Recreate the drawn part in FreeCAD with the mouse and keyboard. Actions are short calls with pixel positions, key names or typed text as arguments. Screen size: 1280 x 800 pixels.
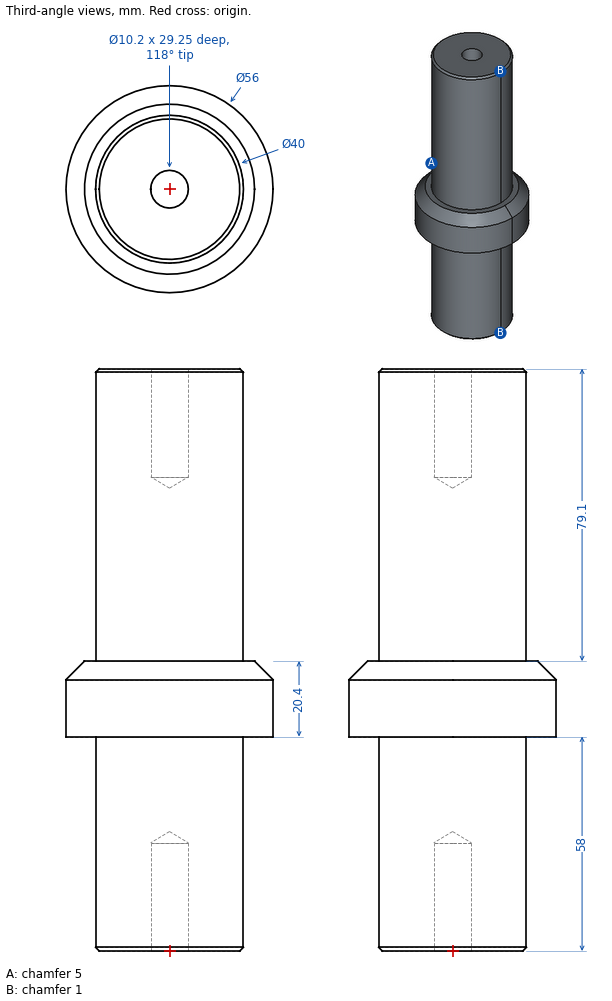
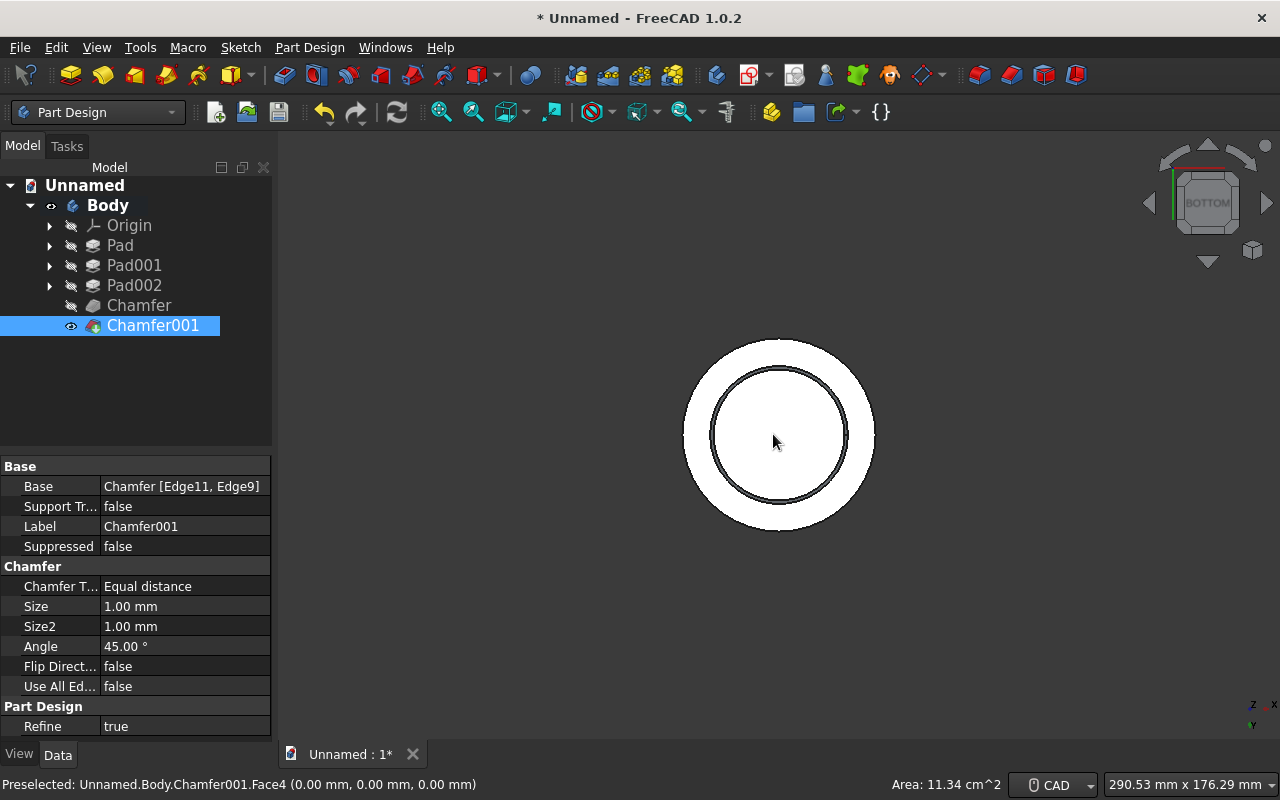
click(750, 76)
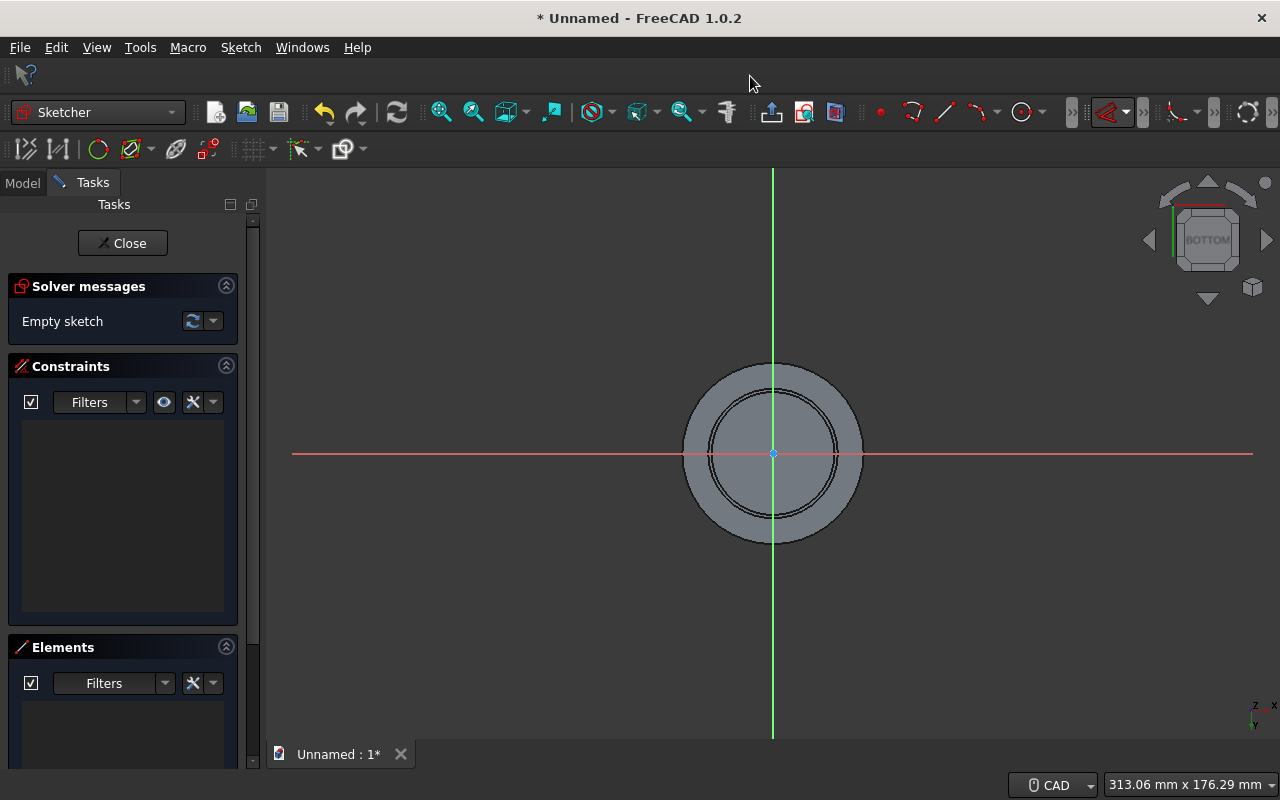
scroll(780, 453, up, 12)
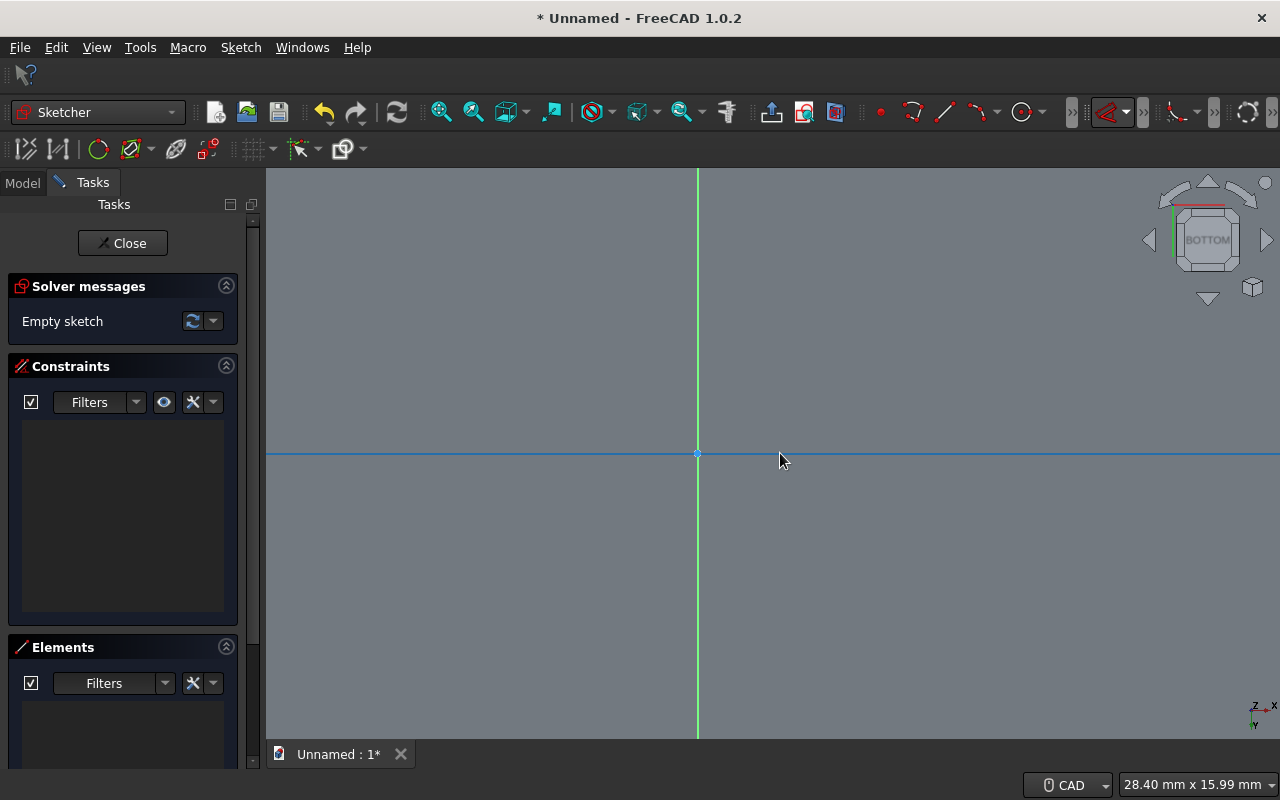
click(1022, 112)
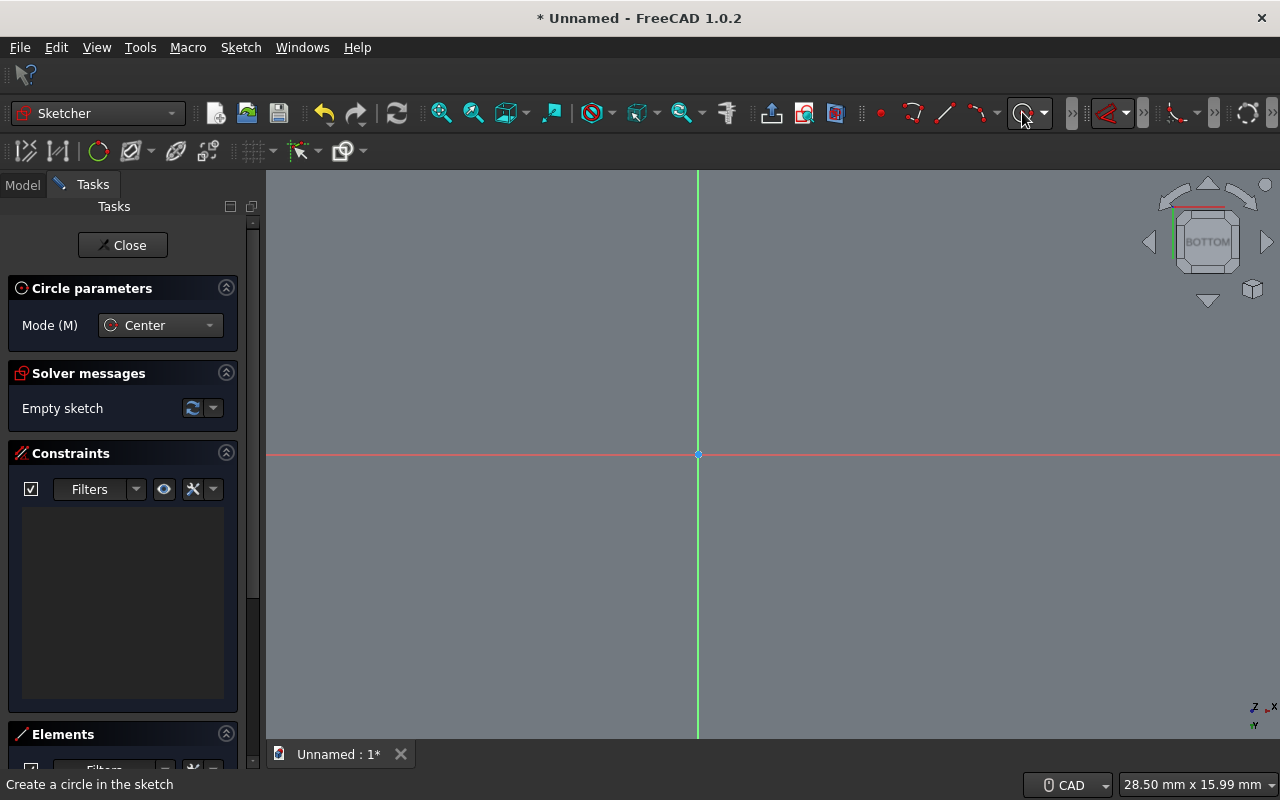
click(698, 454)
move(826, 326)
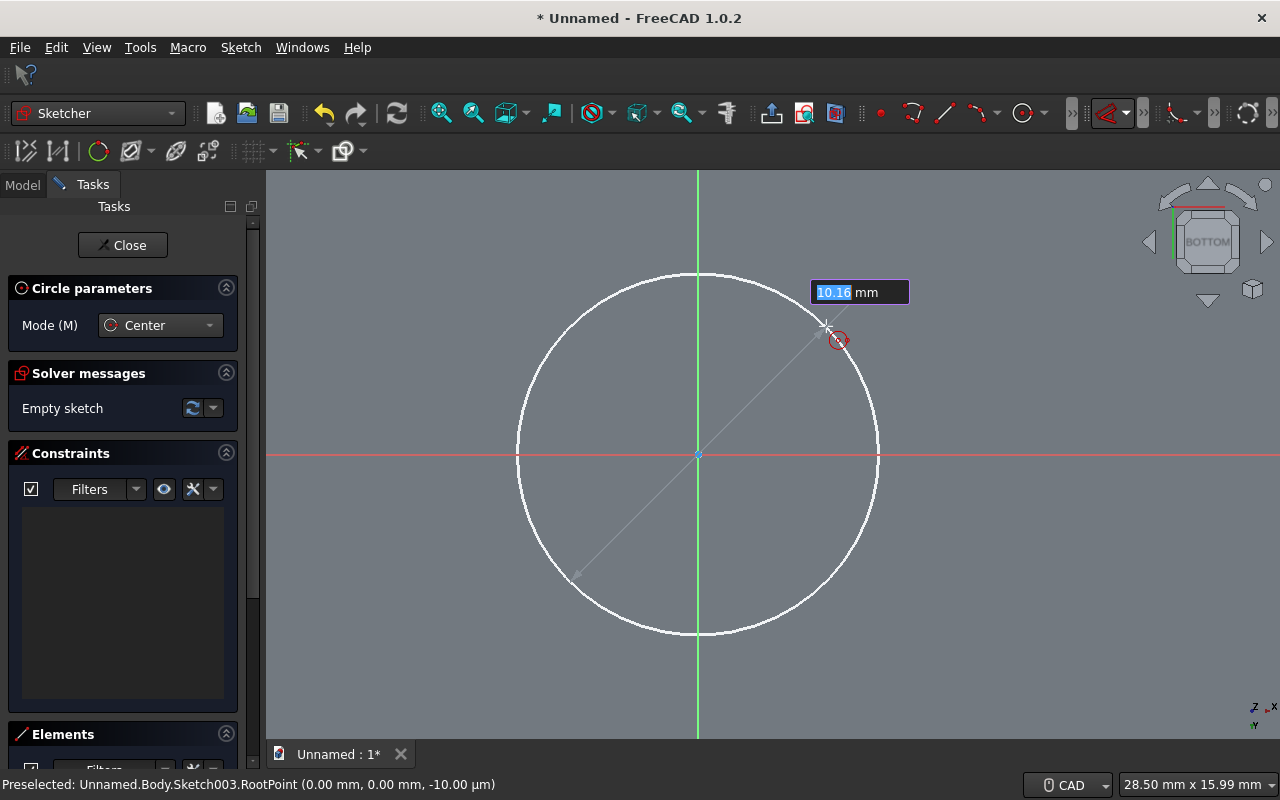
text(10.2)
key(Return)
key(Escape)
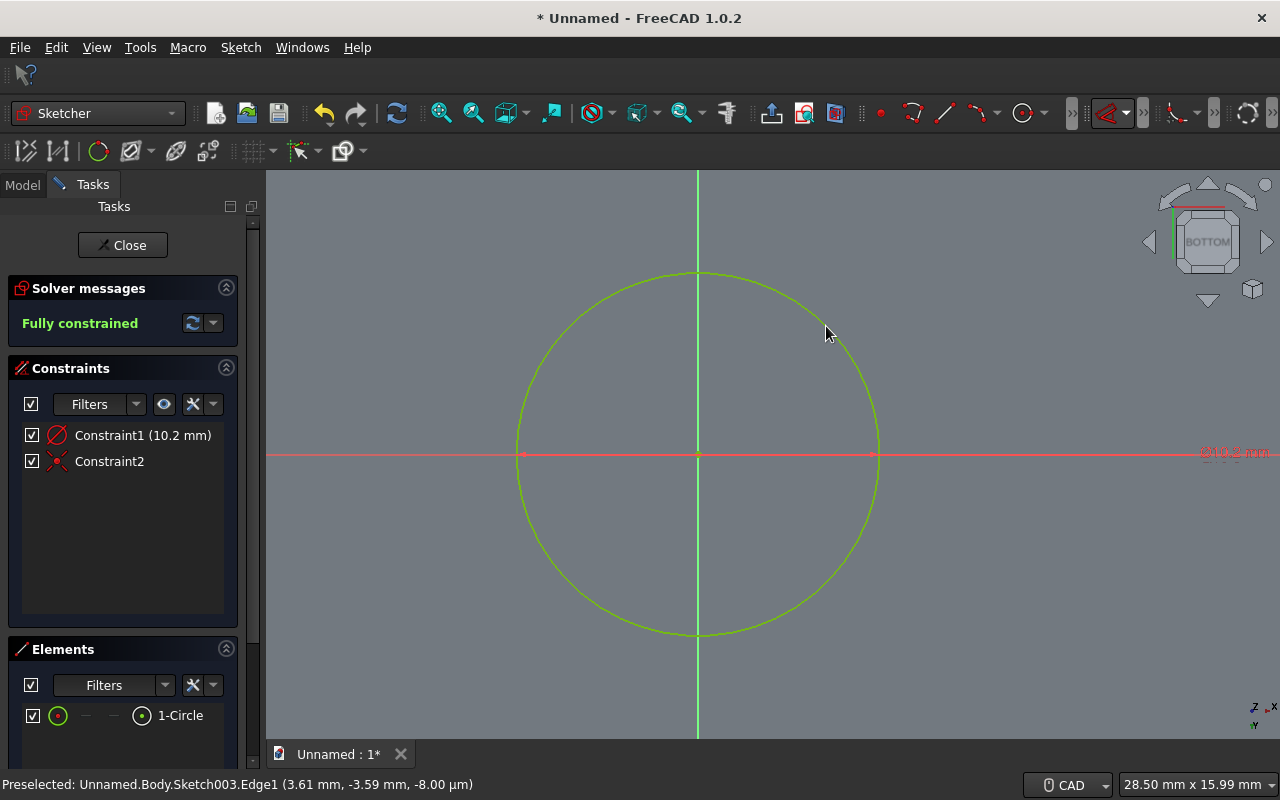
click(123, 245)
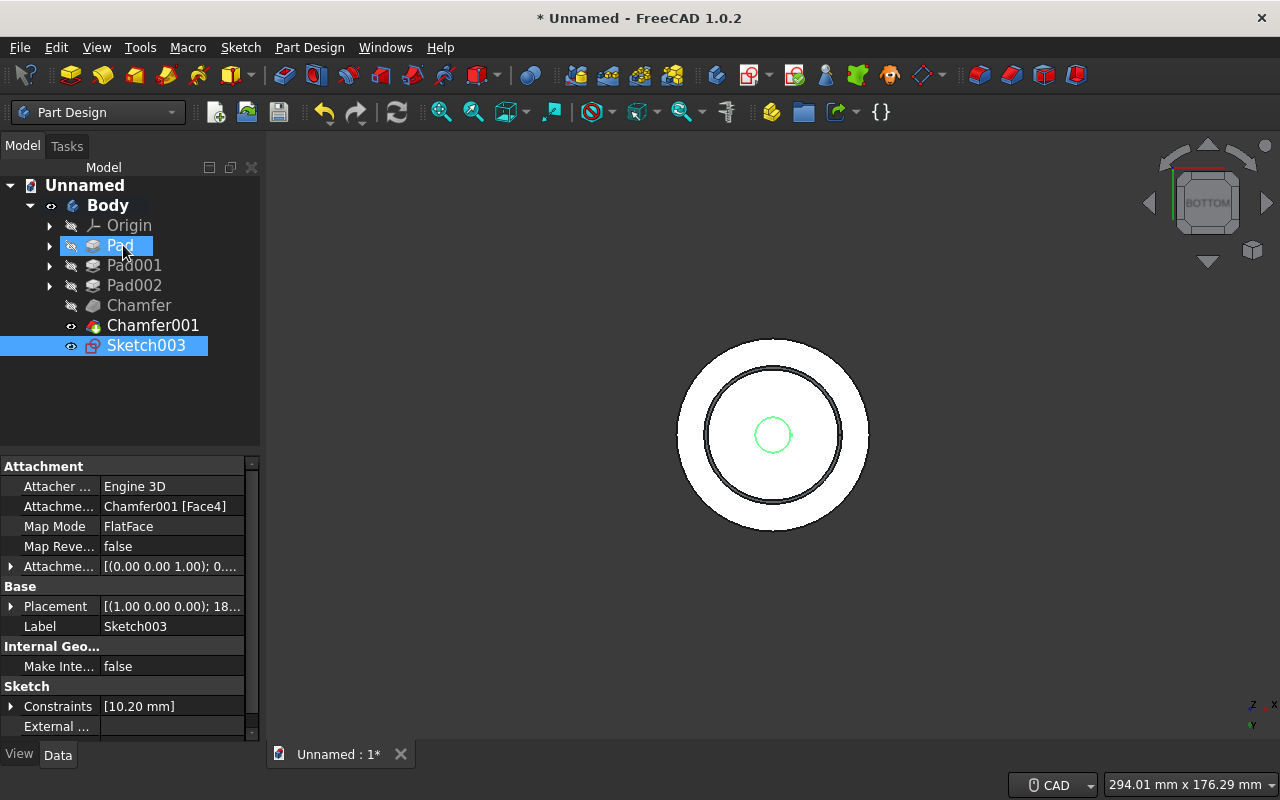
click(318, 76)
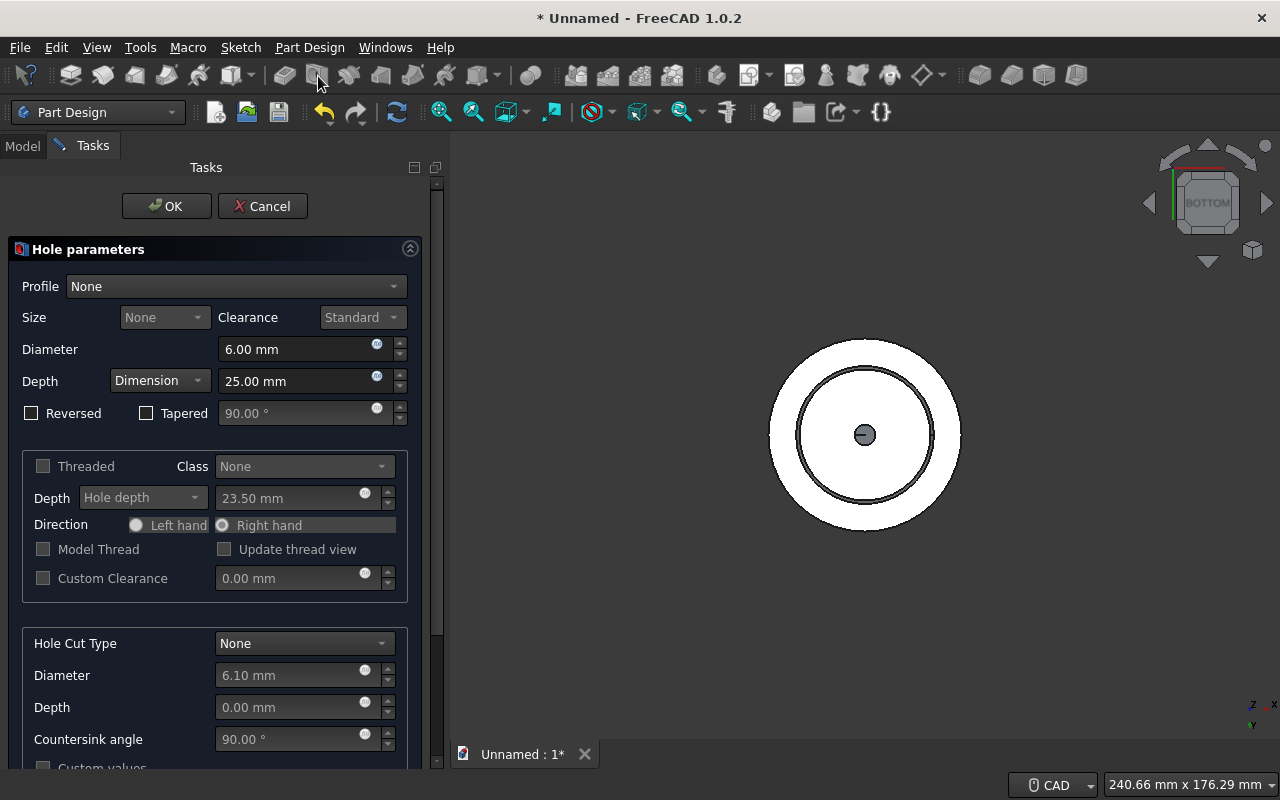
triple_click(305, 349)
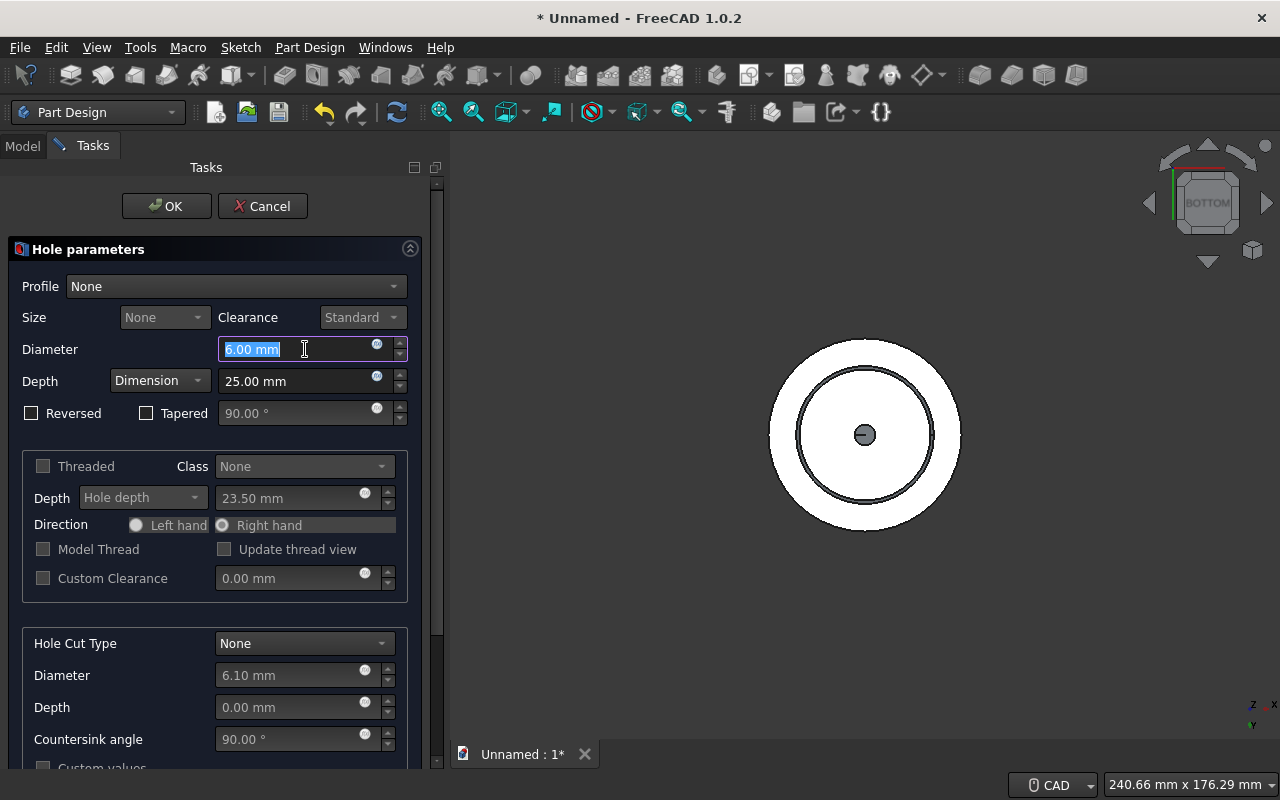
text(10.2)
key(Tab)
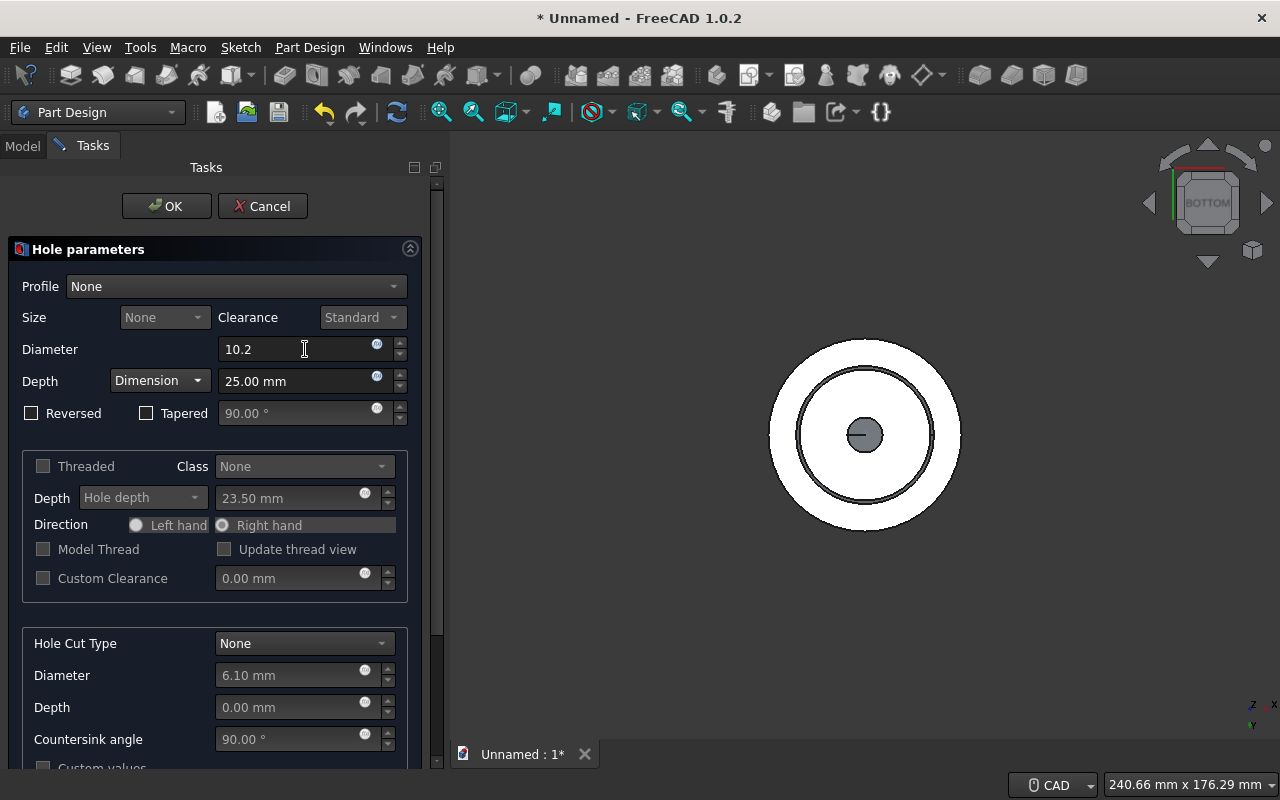
triple_click(305, 381)